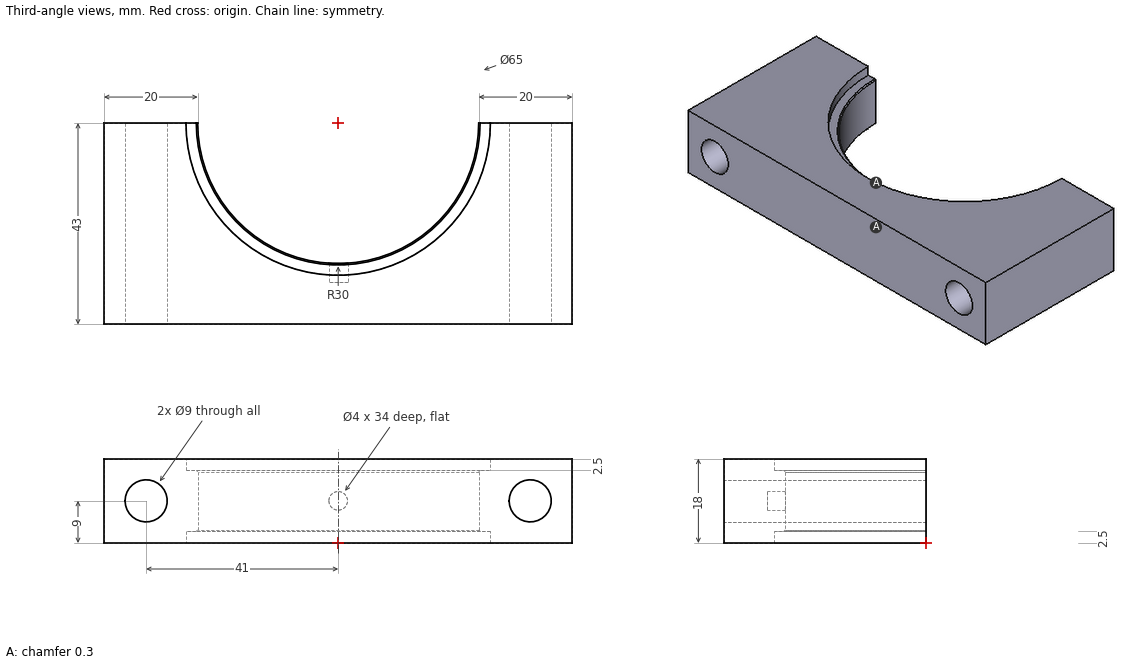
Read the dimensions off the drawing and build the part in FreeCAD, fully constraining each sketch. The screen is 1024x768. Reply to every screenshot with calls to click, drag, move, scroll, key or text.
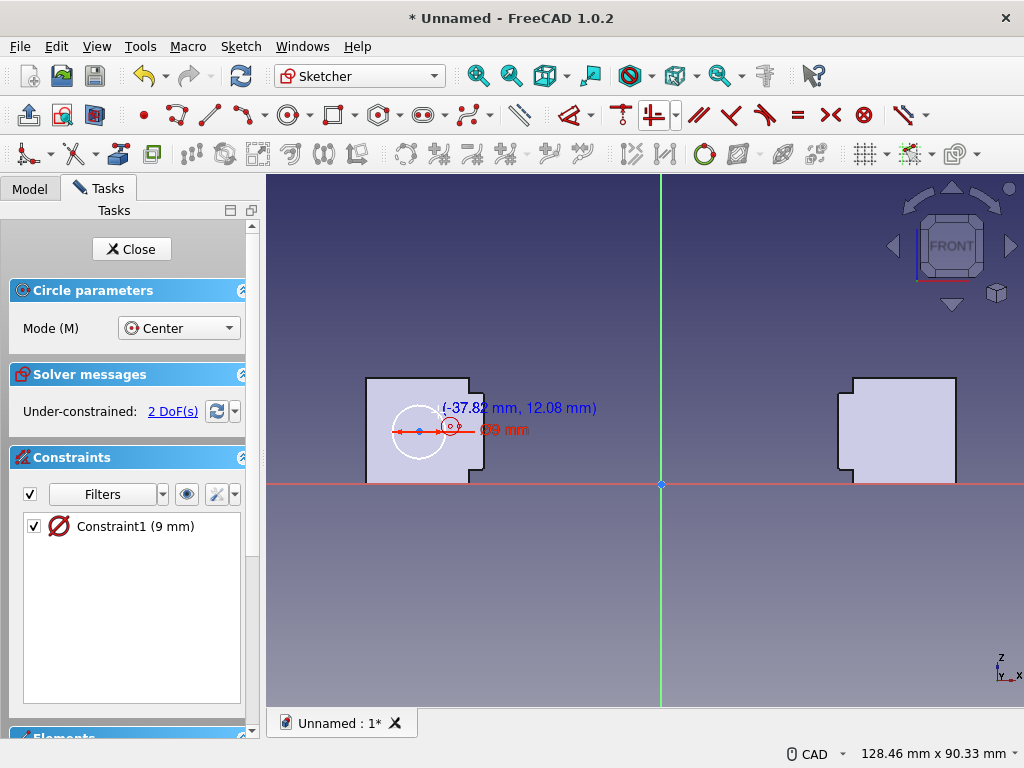
scroll(294, 423, down, 1)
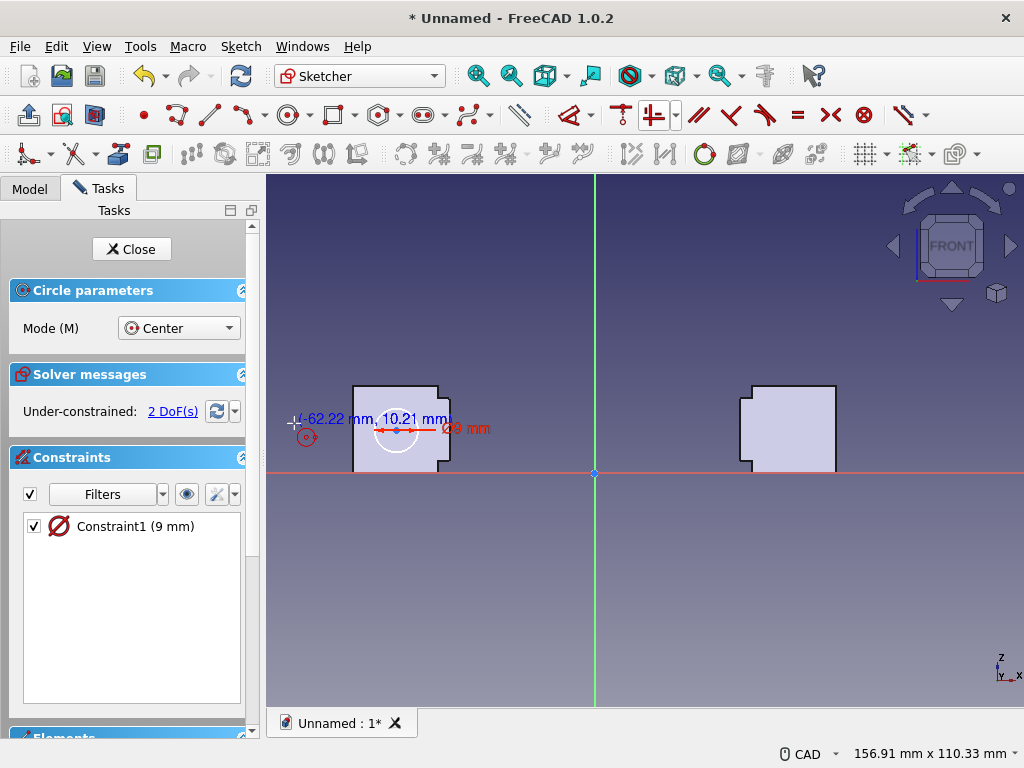
click(793, 430)
move(808, 414)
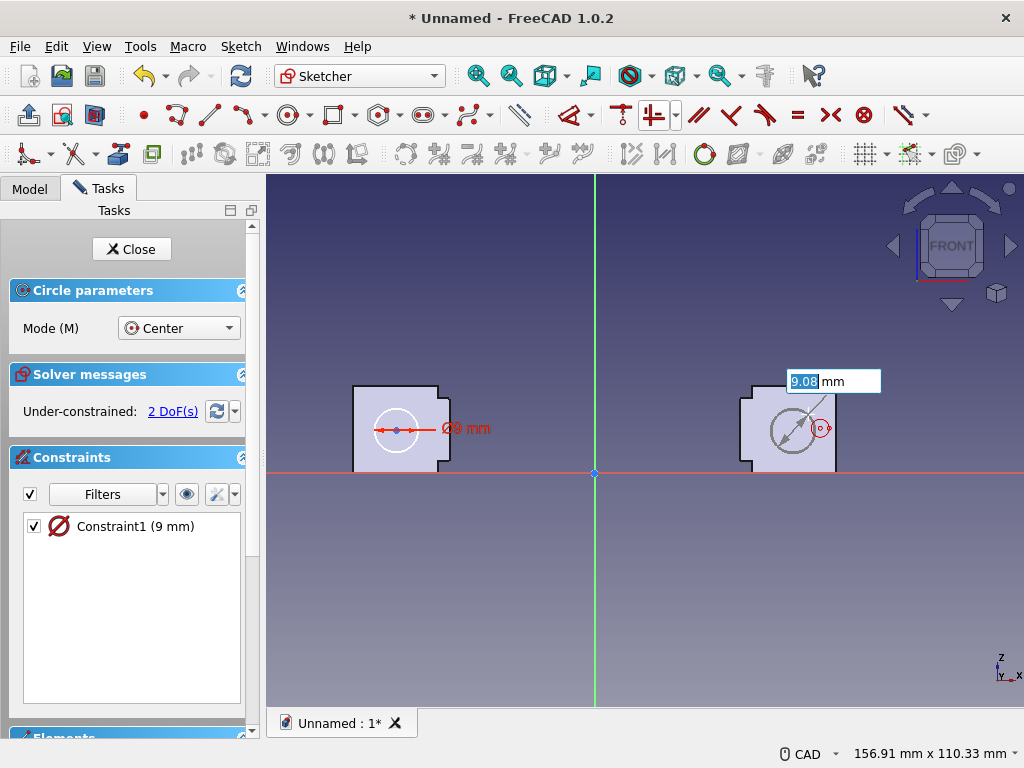
text(9)
key(Return)
key(Escape)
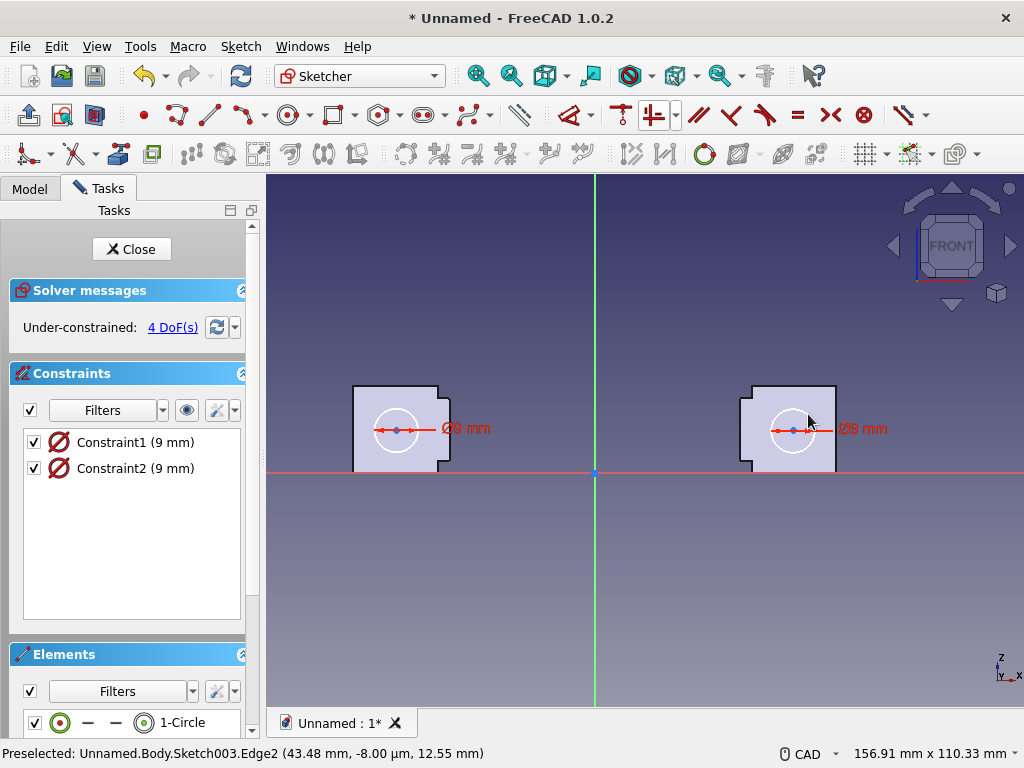
click(396, 430)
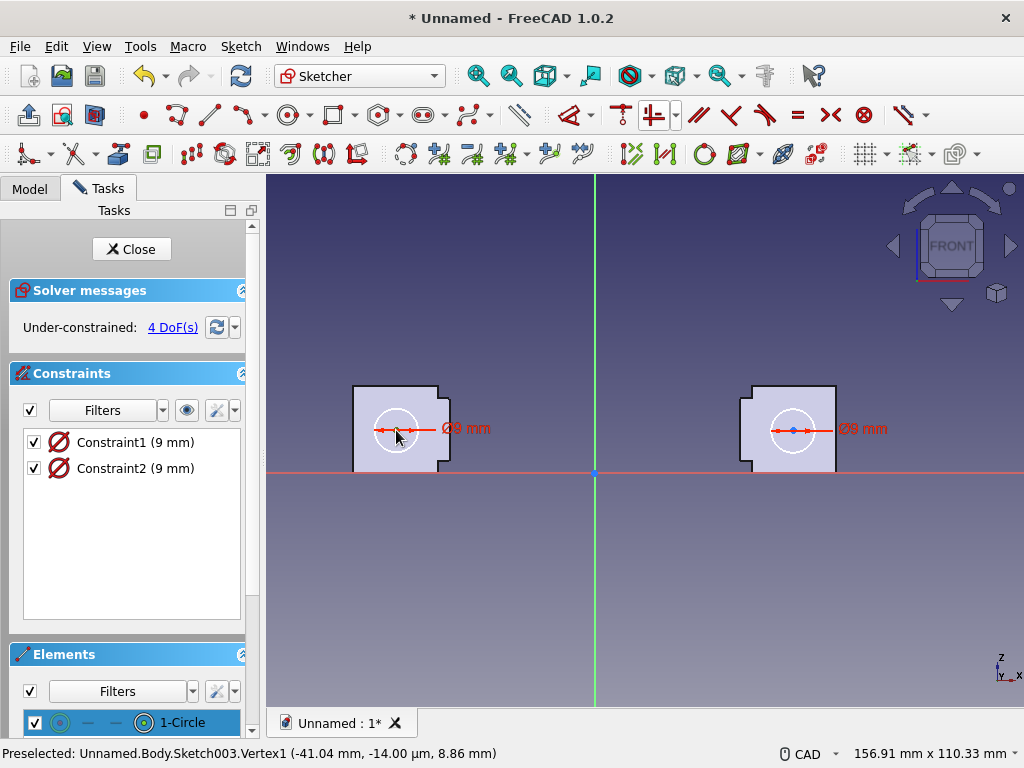
click(793, 431)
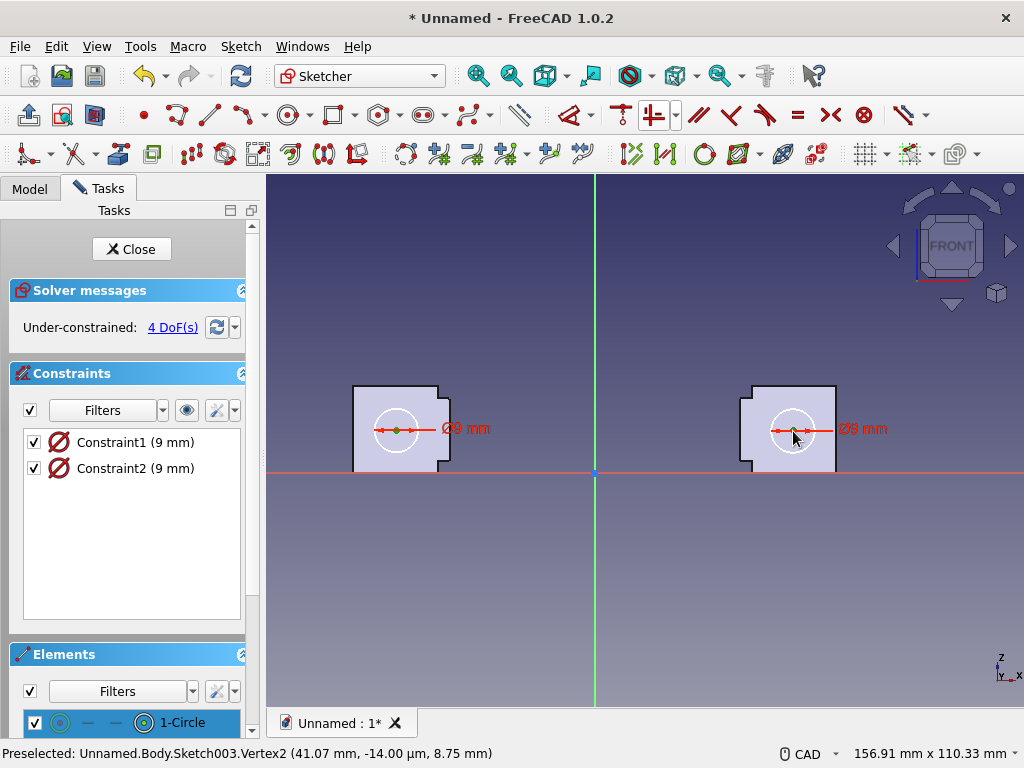
click(595, 645)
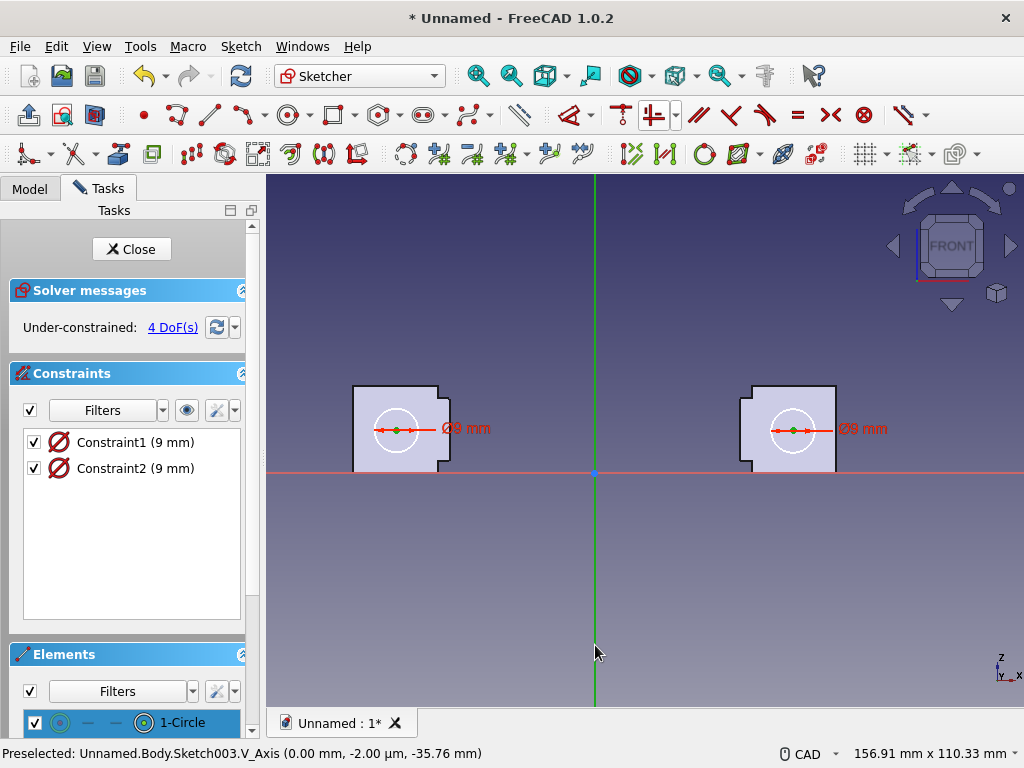
click(831, 116)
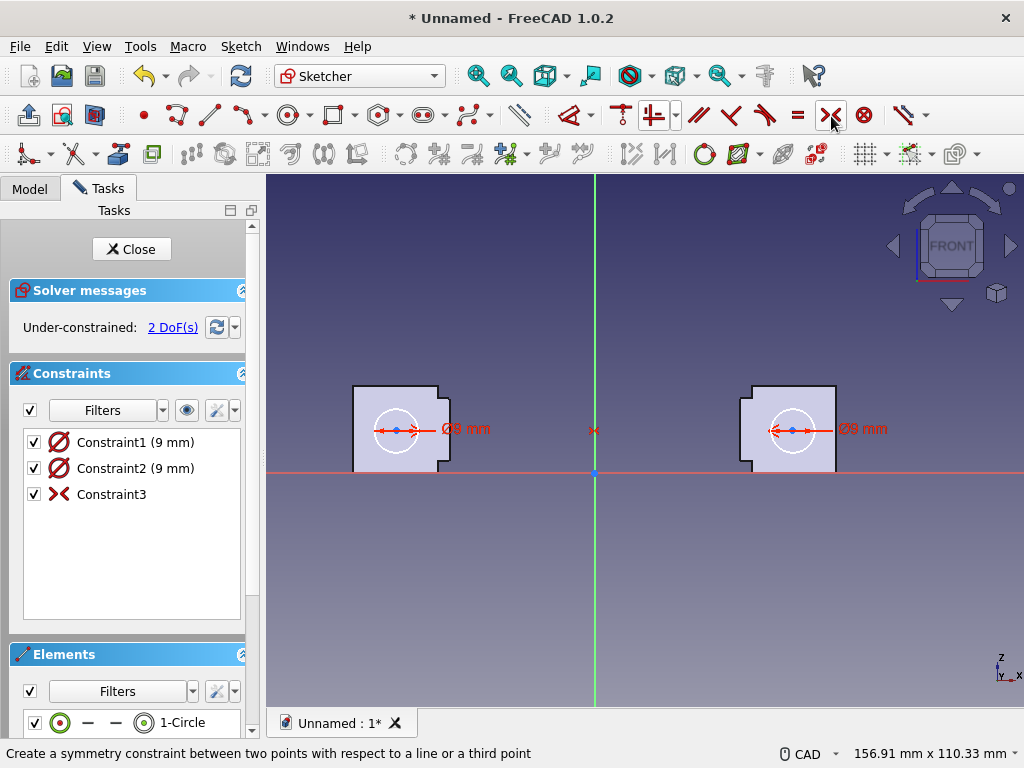
click(568, 116)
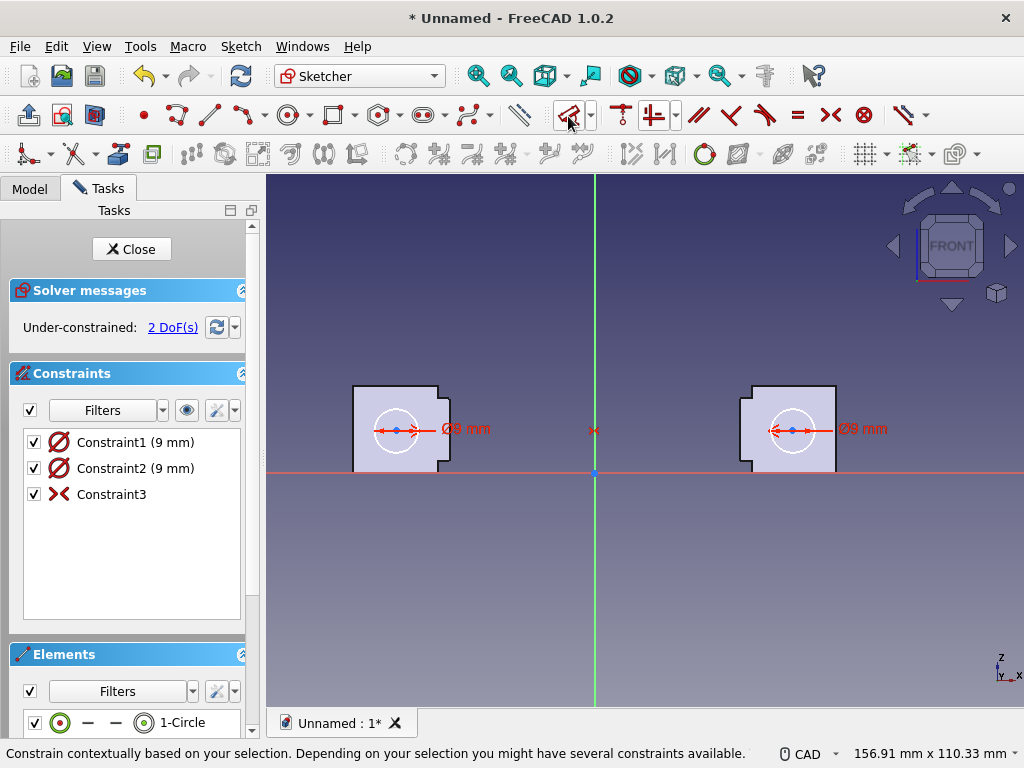
click(396, 431)
click(362, 452)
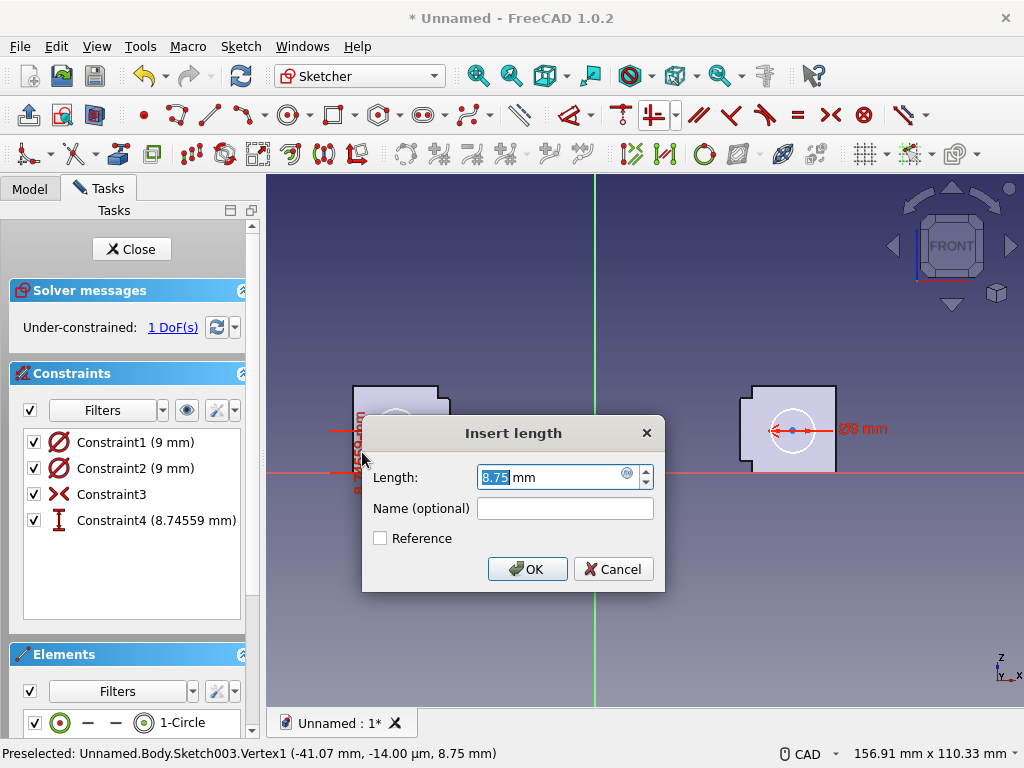
text(9)
key(Return)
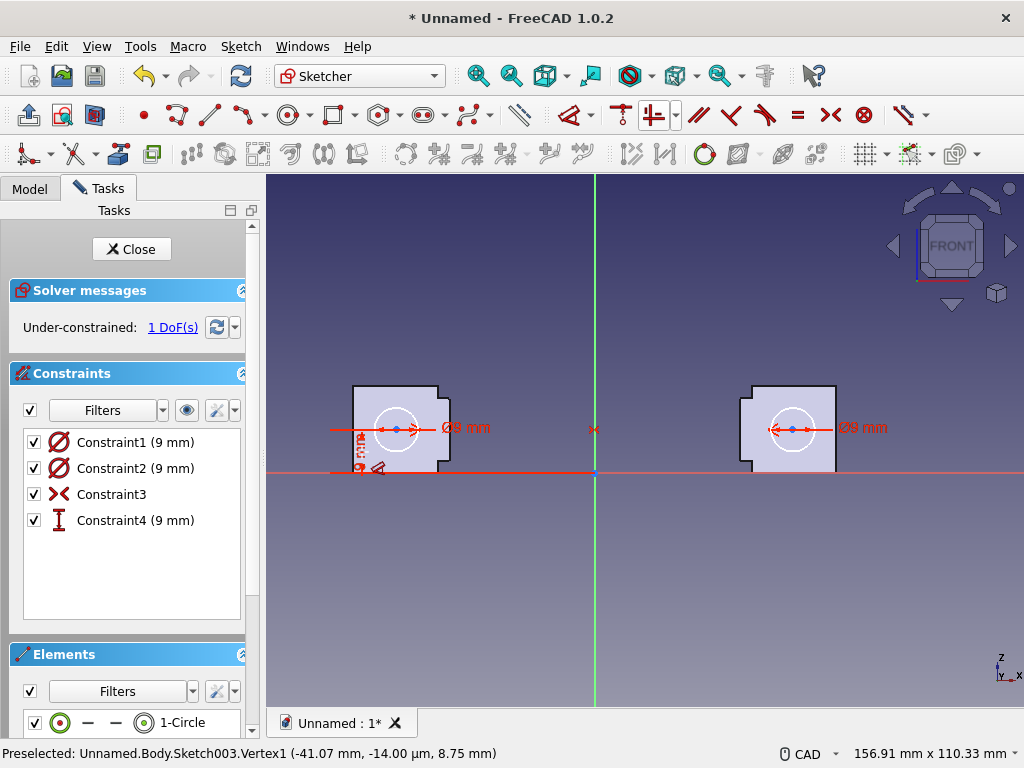
click(396, 430)
click(495, 507)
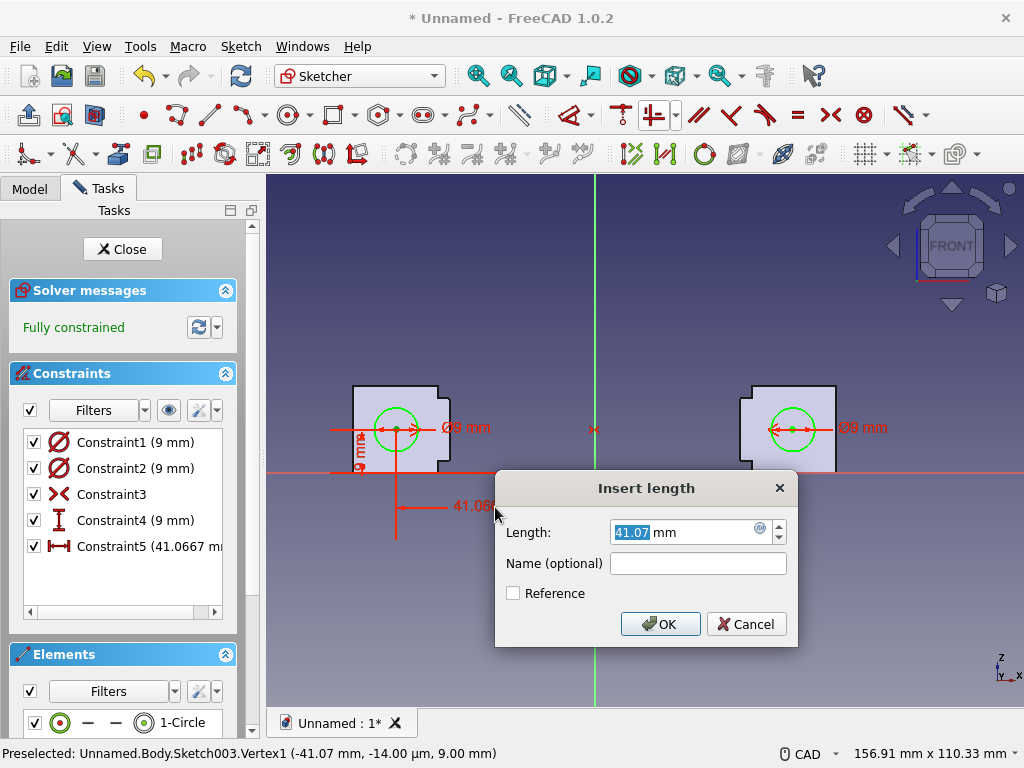
text(41)
key(Return)
key(Escape)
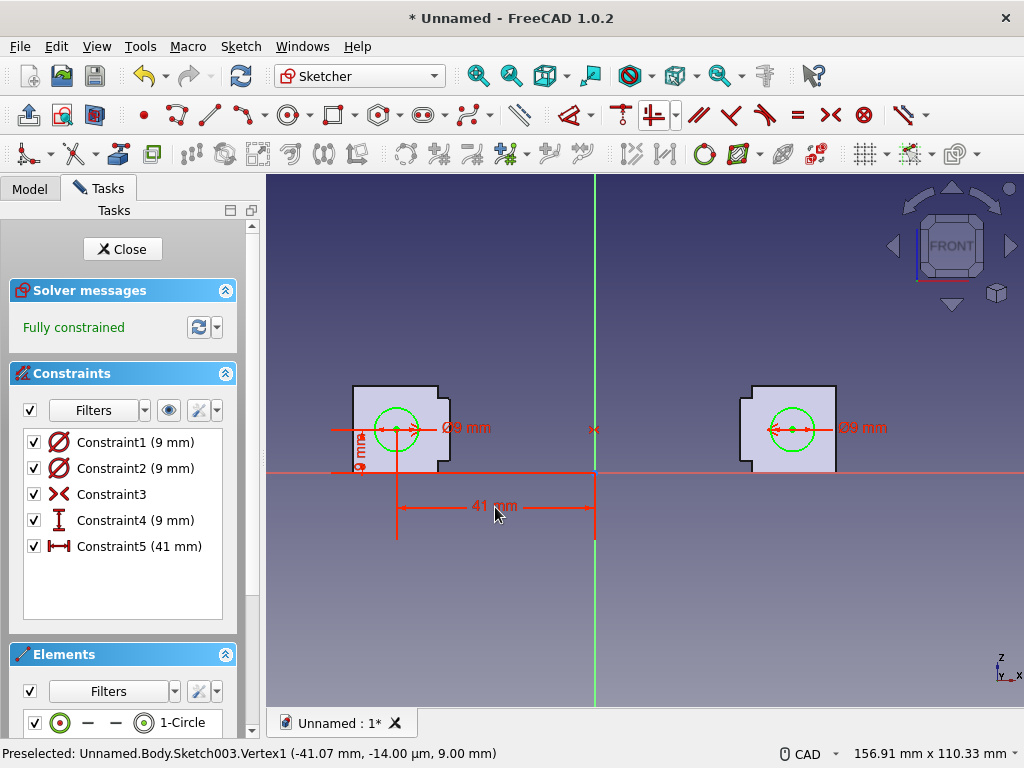
click(123, 249)